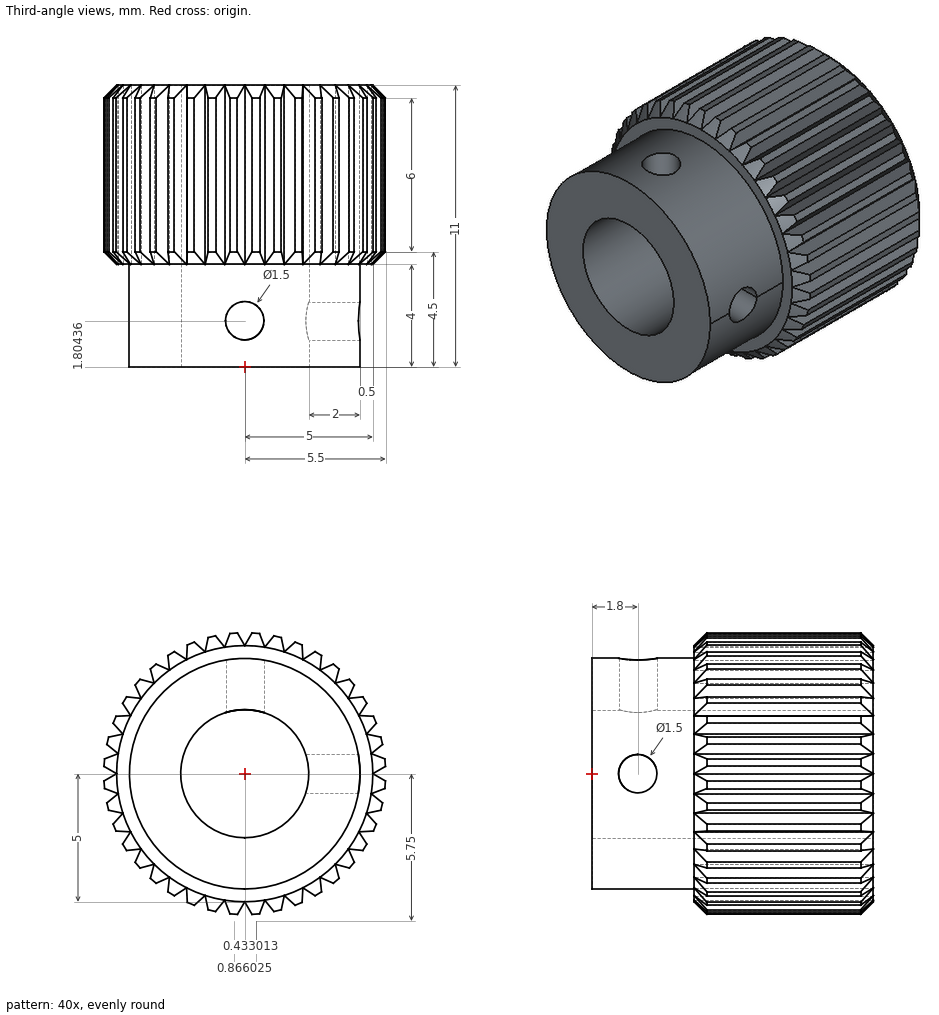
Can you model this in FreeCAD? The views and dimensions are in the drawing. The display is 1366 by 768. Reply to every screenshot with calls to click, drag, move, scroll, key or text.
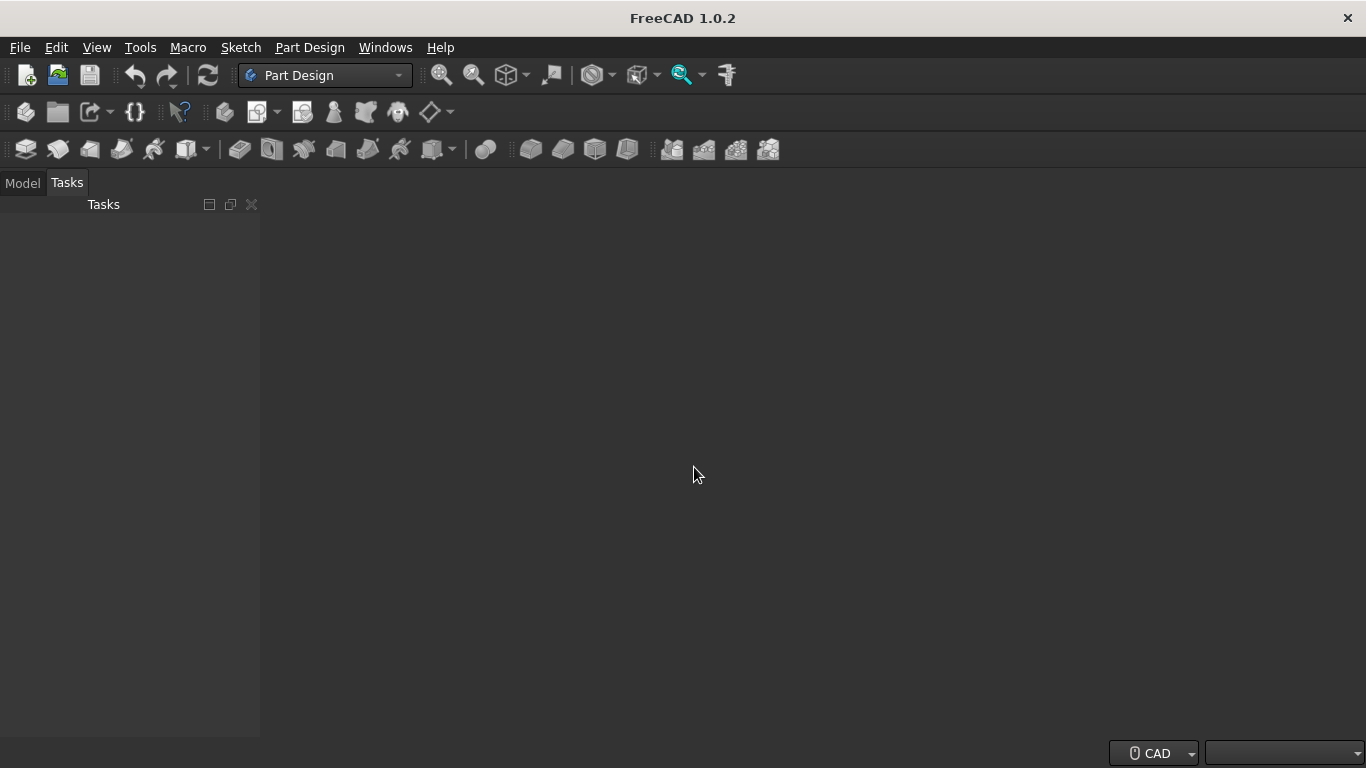
click(26, 76)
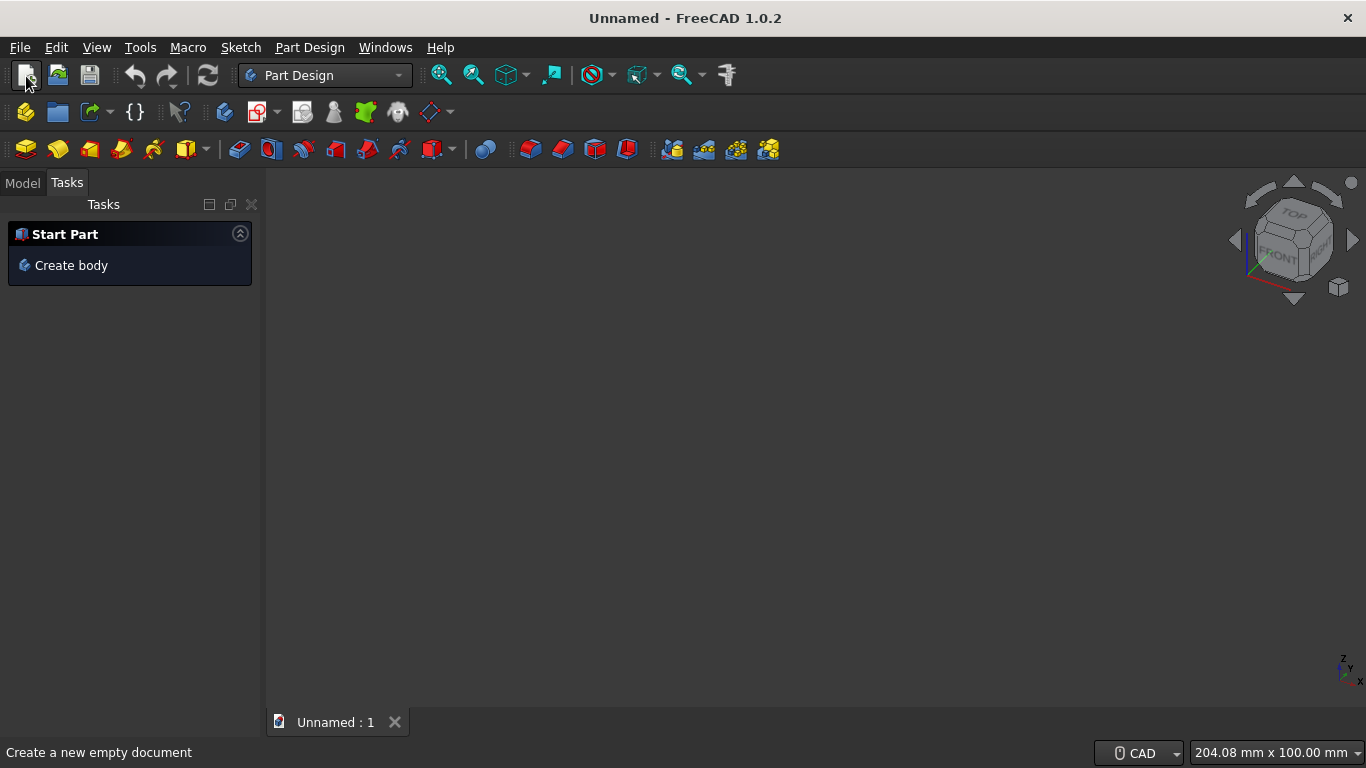
click(258, 112)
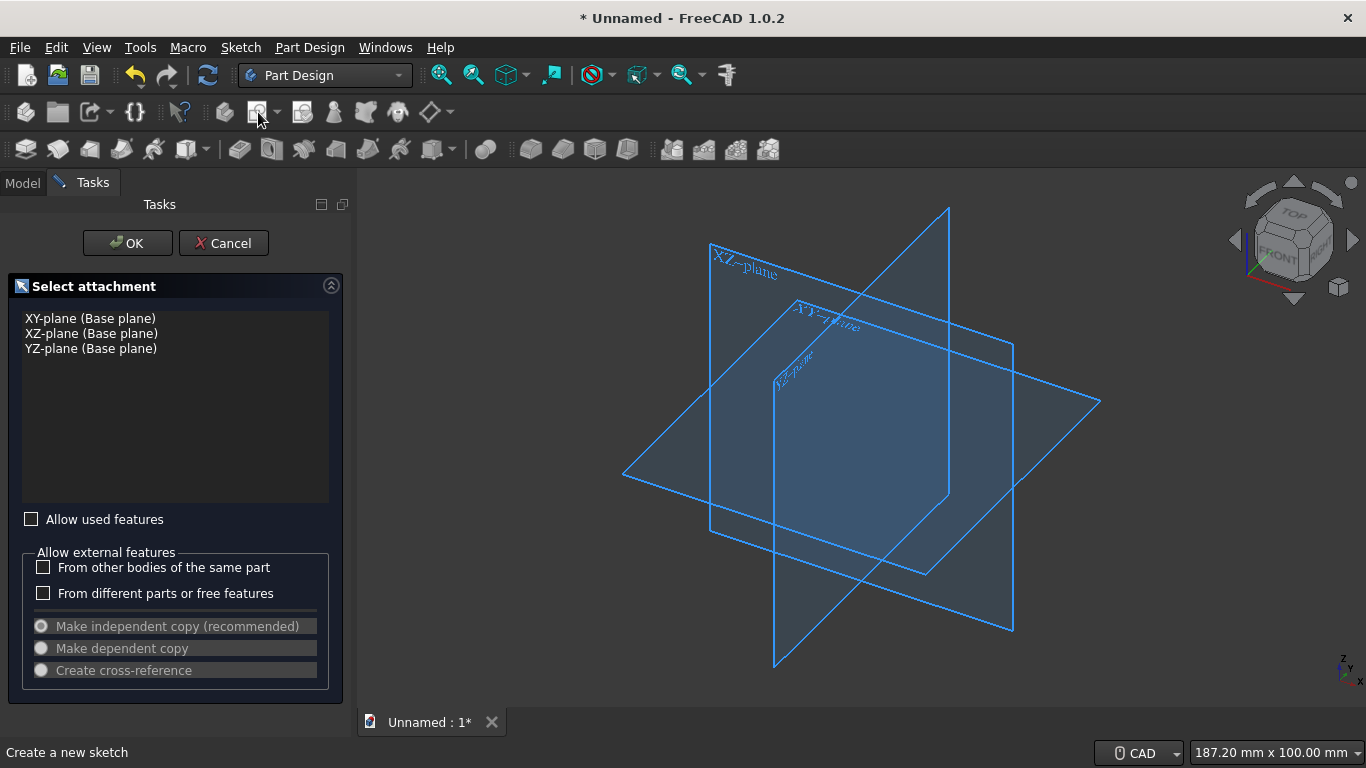
click(82, 318)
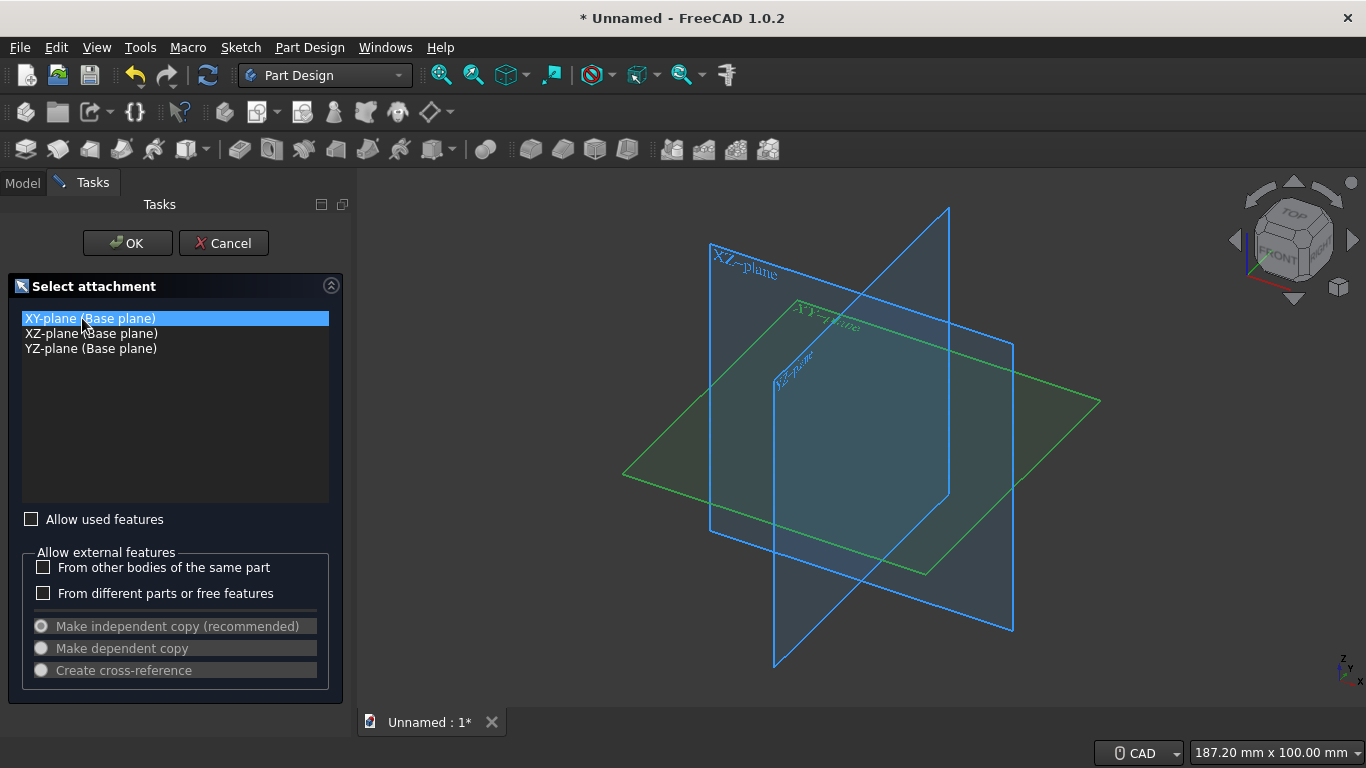
click(128, 243)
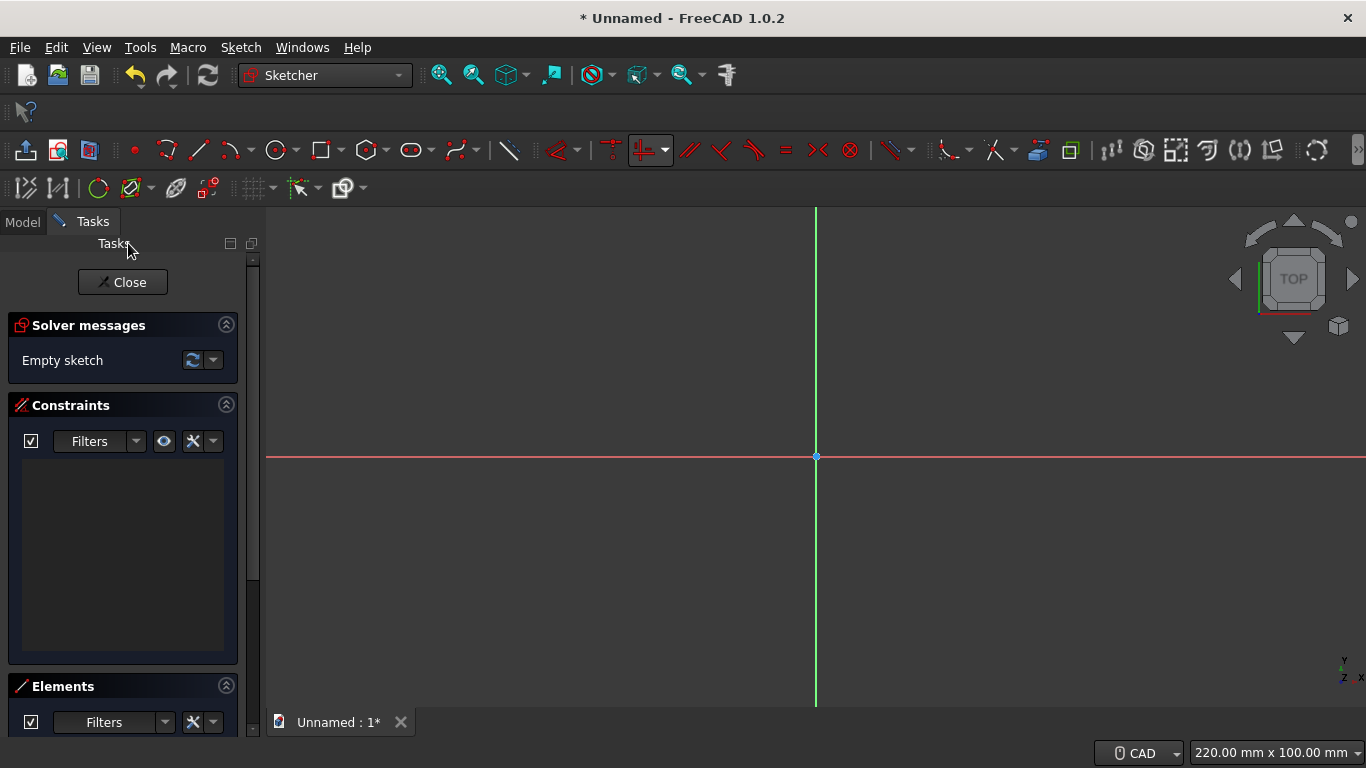
scroll(846, 424, up, 9)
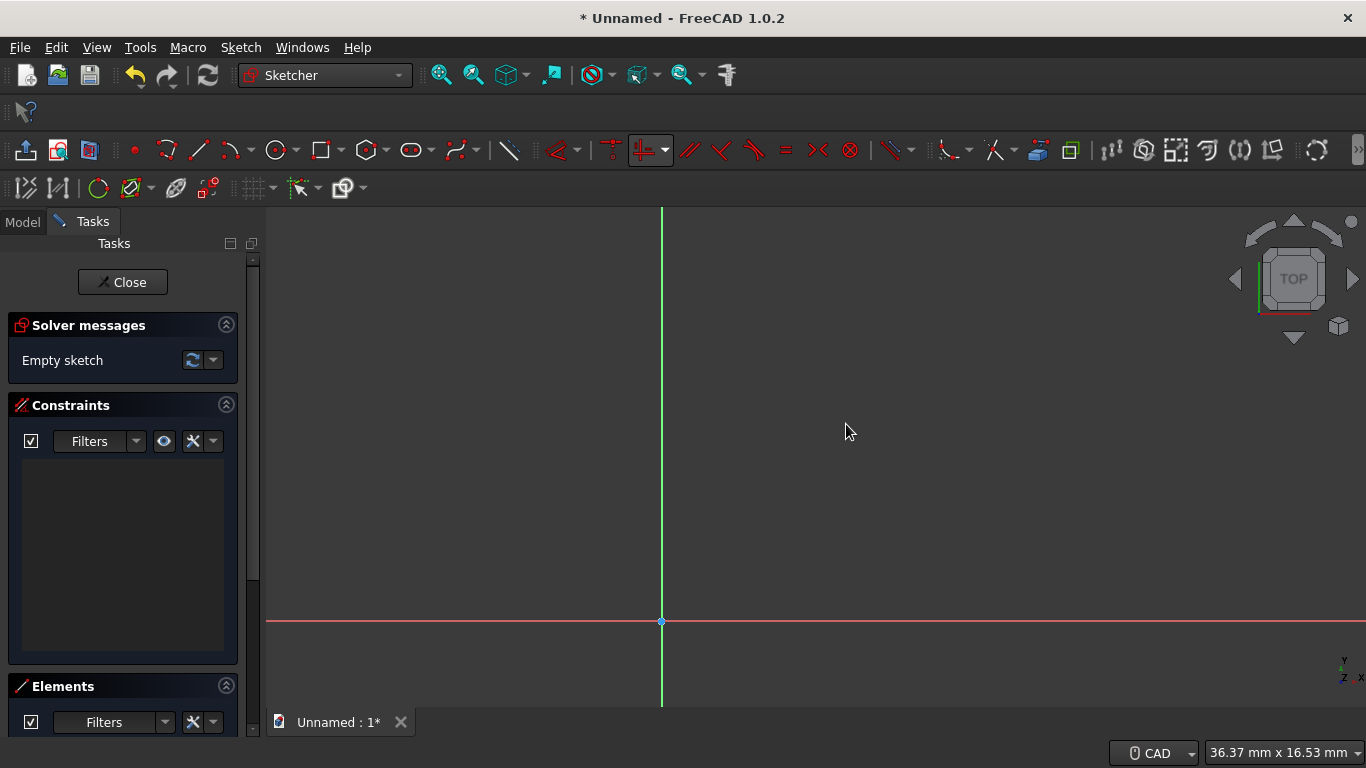
key(g)
key(m)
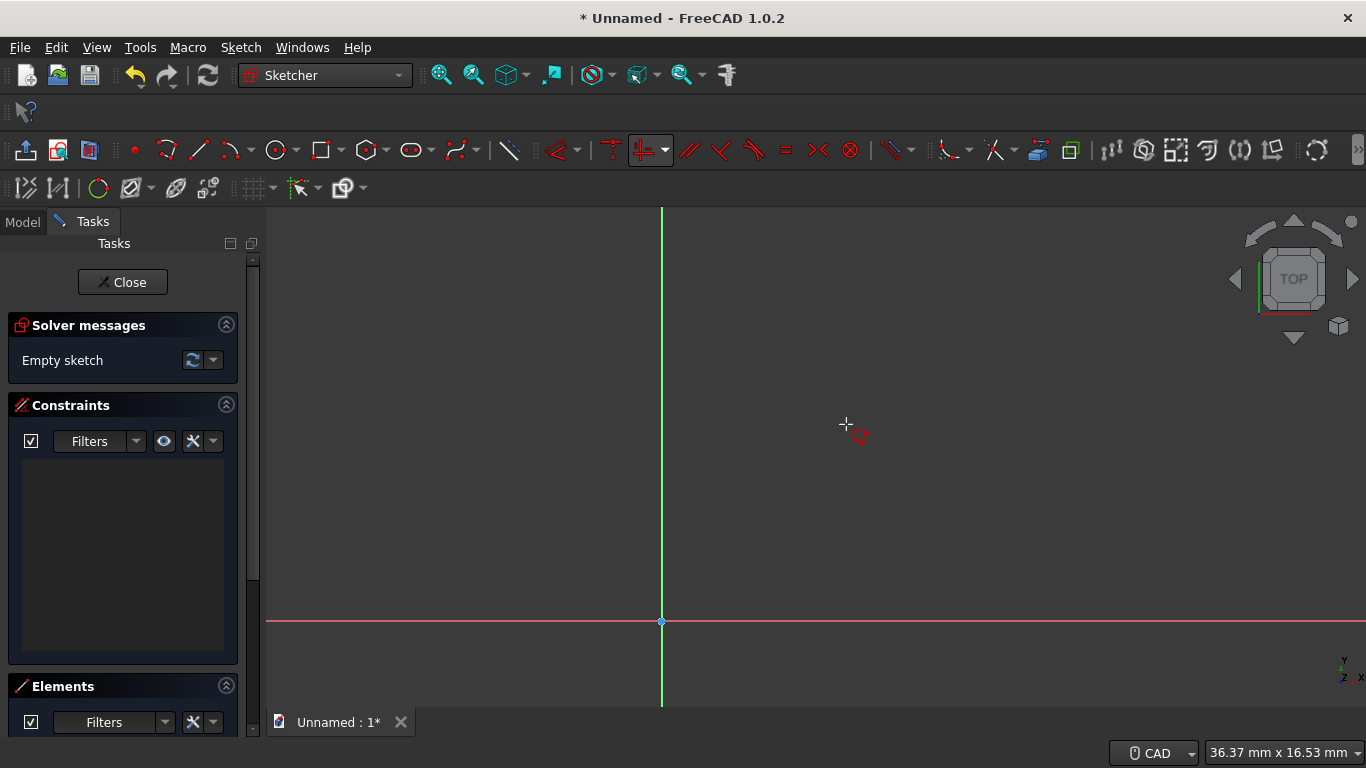
click(737, 621)
click(798, 612)
click(798, 500)
click(813, 500)
click(828, 485)
click(828, 304)
click(813, 289)
click(737, 289)
click(737, 621)
key(Escape)
key(Escape)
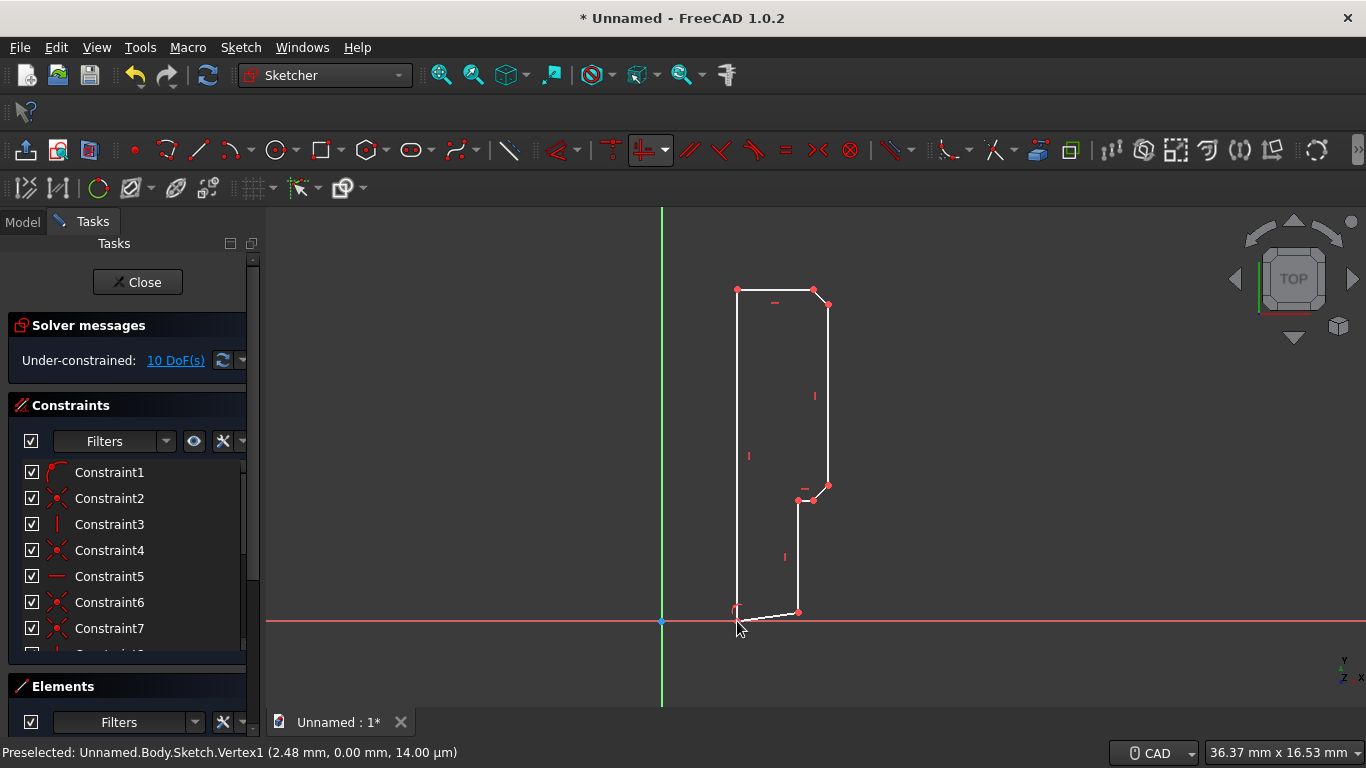
click(755, 619)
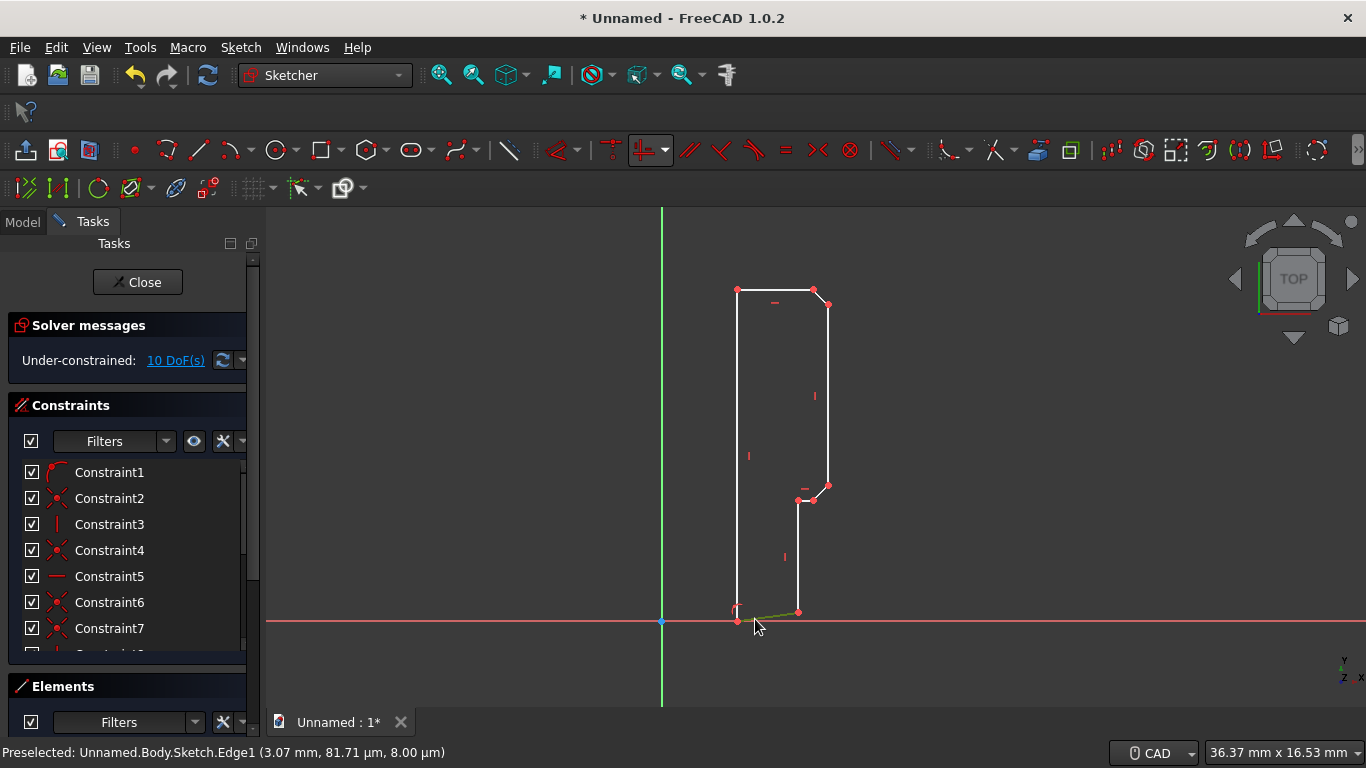
key(h)